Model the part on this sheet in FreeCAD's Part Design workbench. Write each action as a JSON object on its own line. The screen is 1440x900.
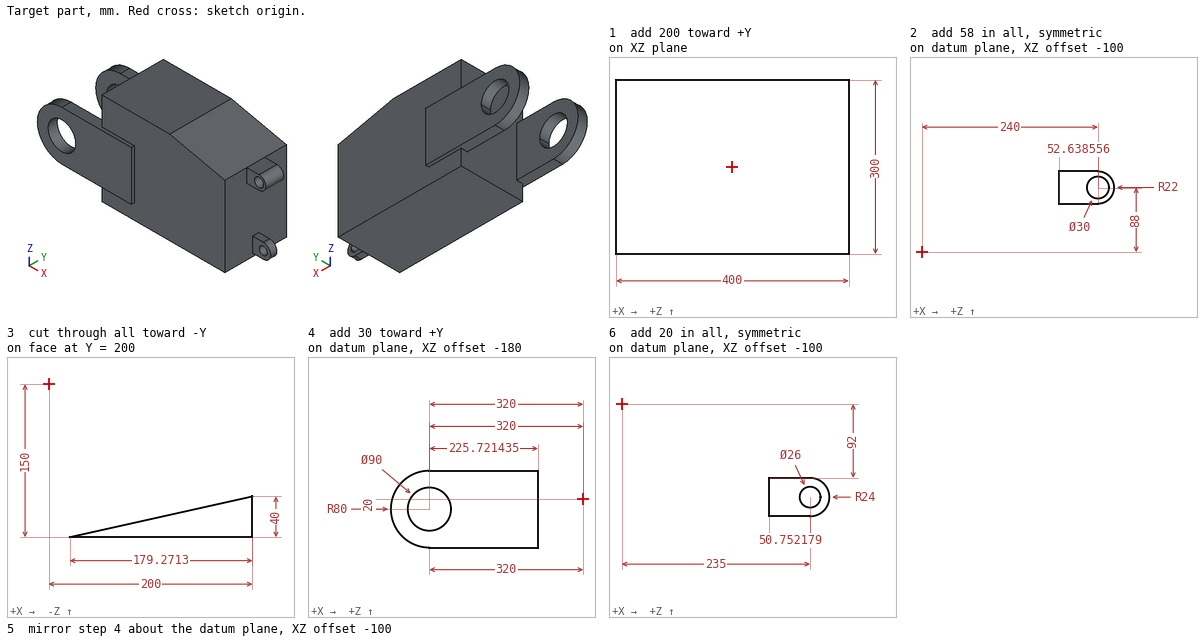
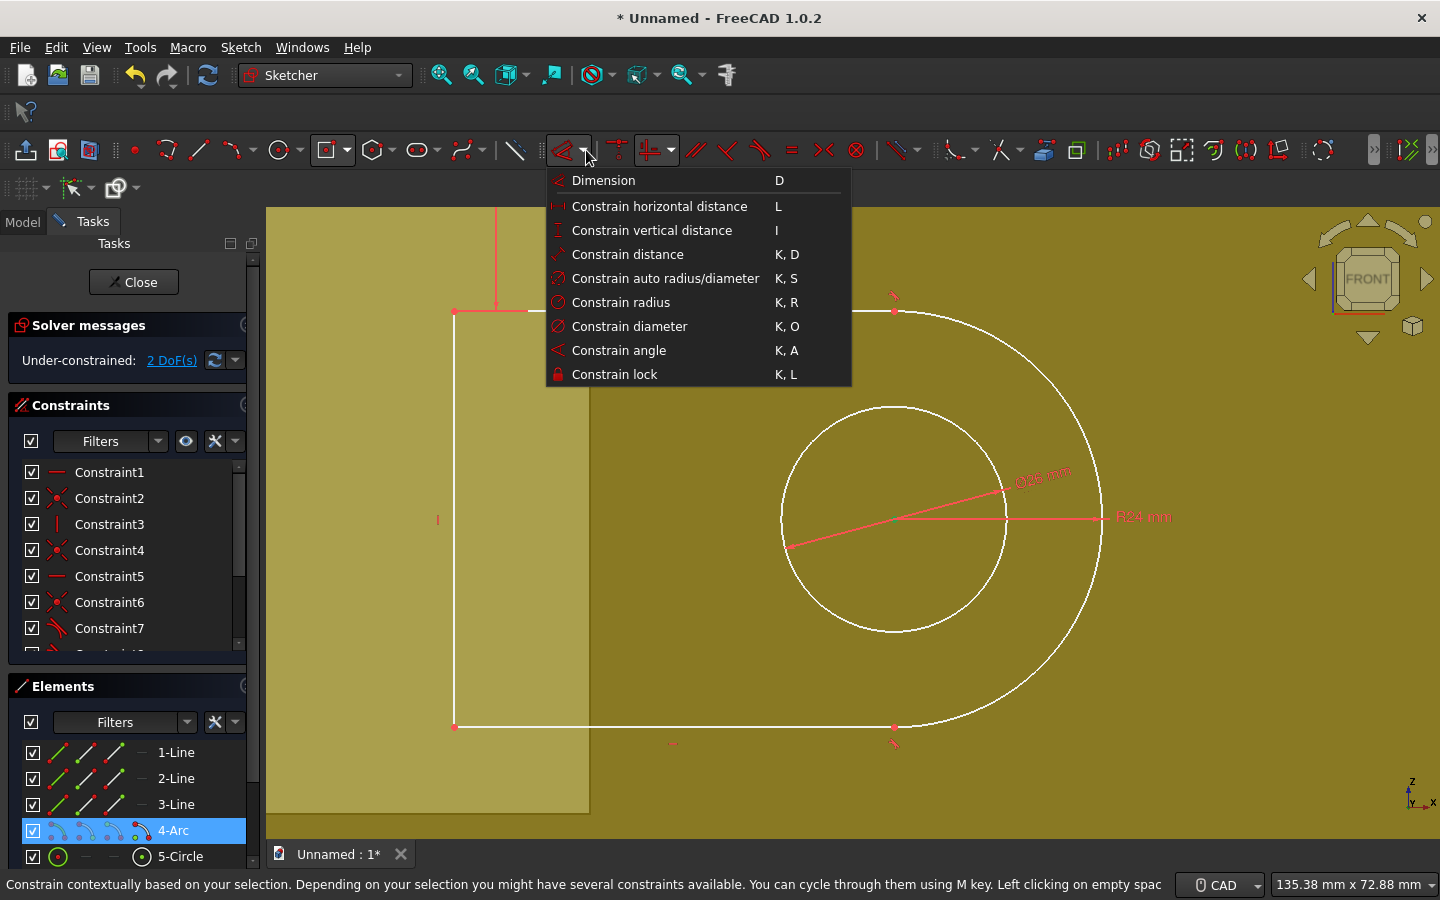
{"action": "left_click", "coordinate": [699, 206]}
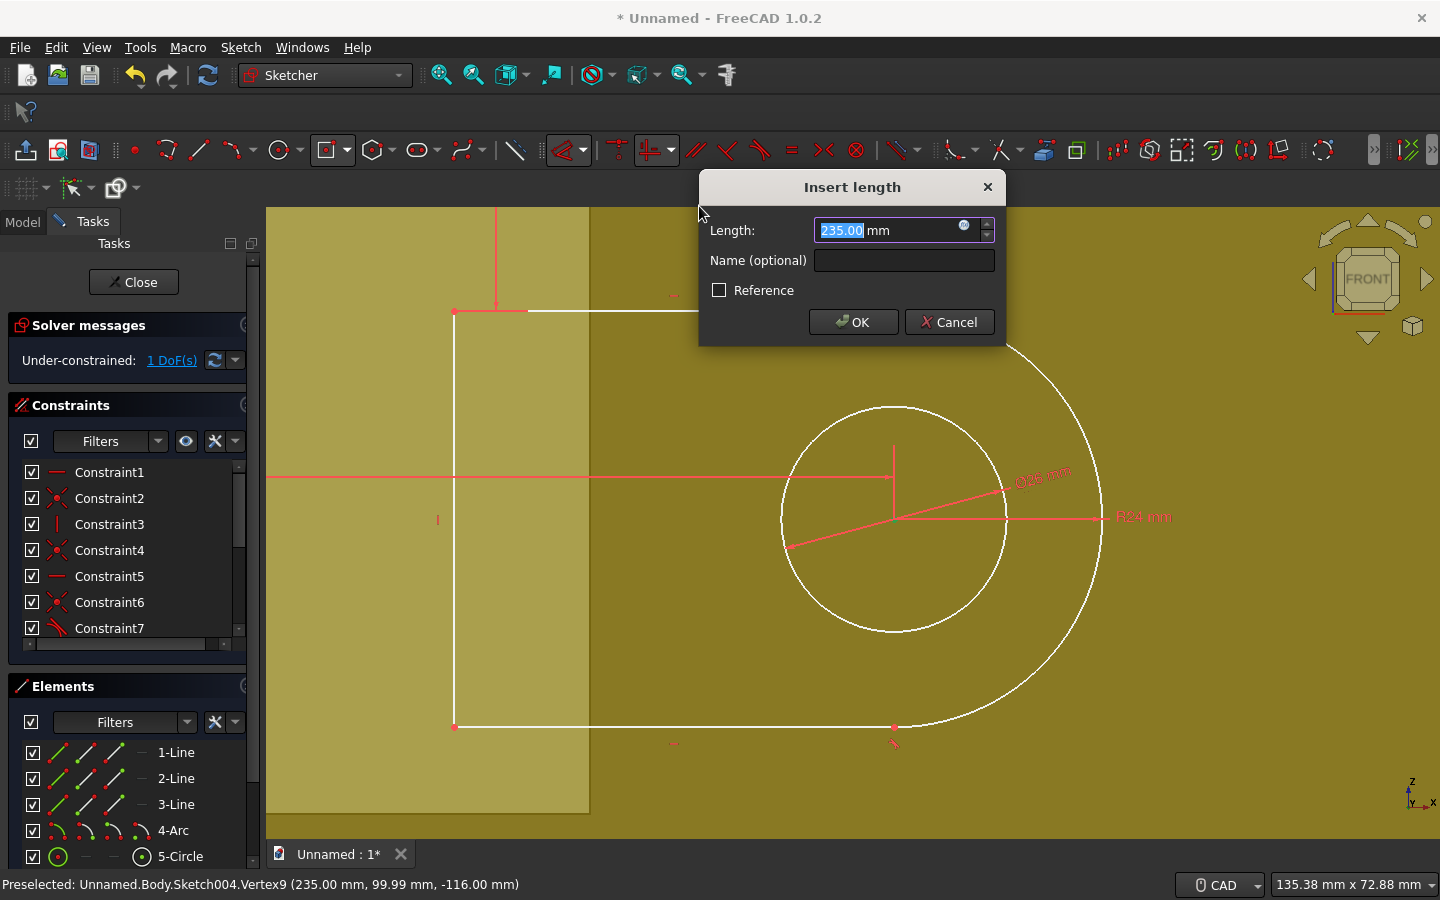
{"action": "type", "text": "235"}
{"action": "key", "text": "Return"}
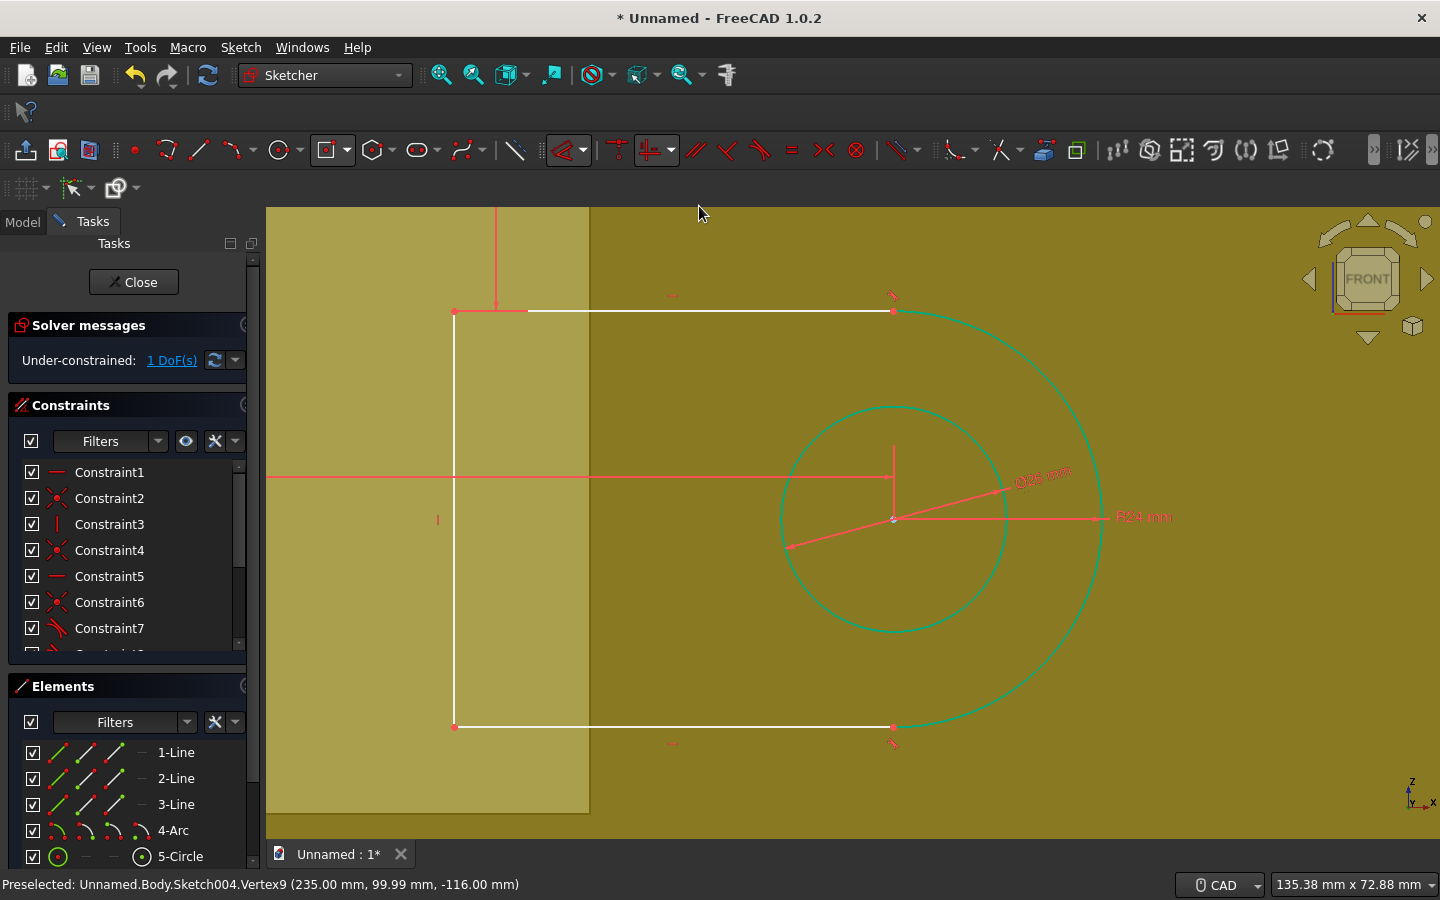
{"action": "left_click", "coordinate": [762, 727]}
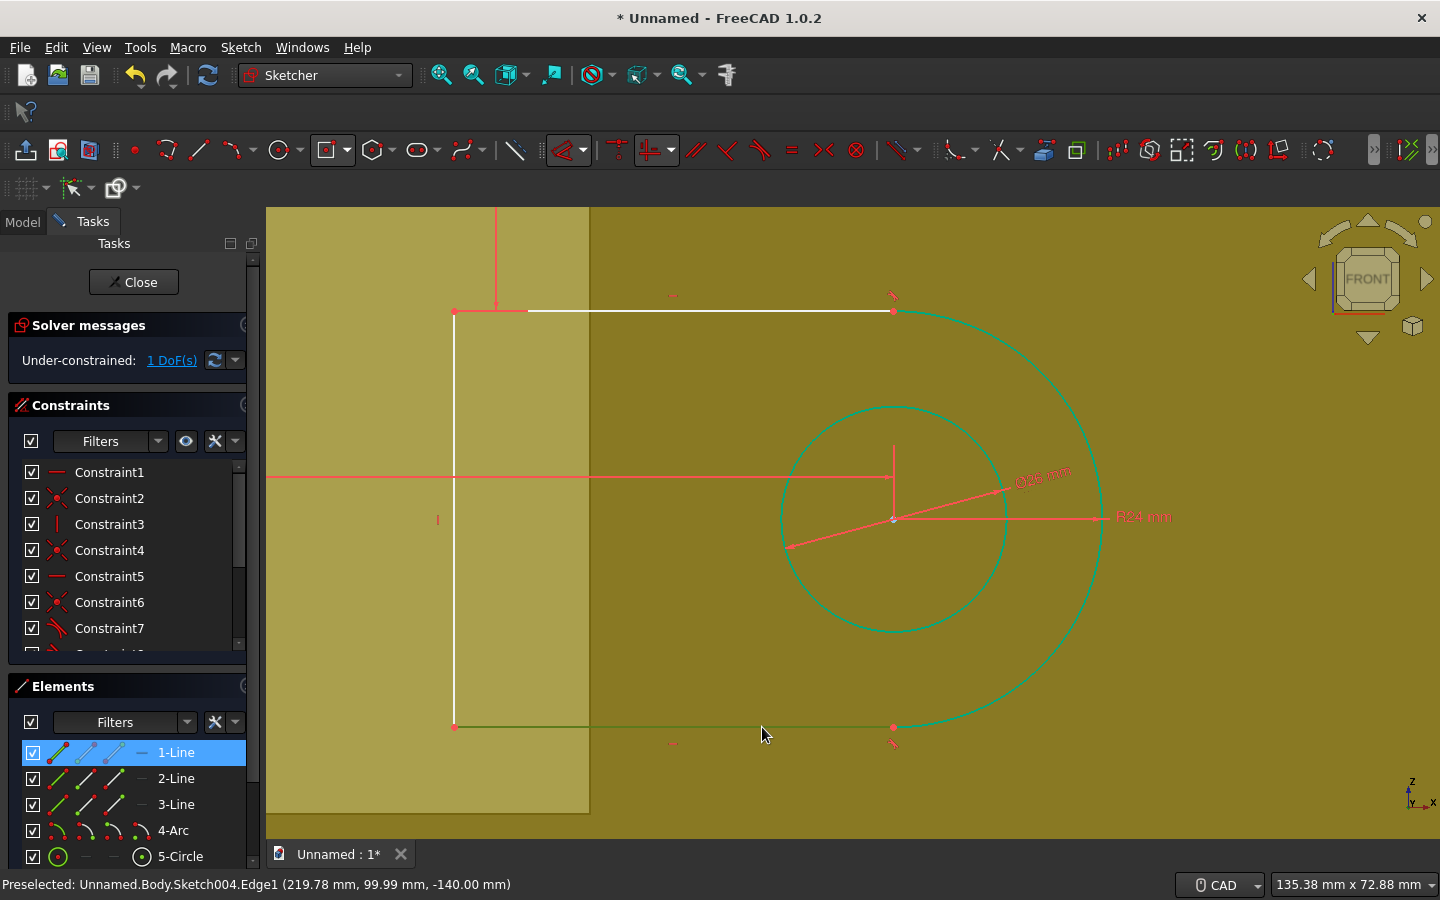
{"action": "key", "text": "l"}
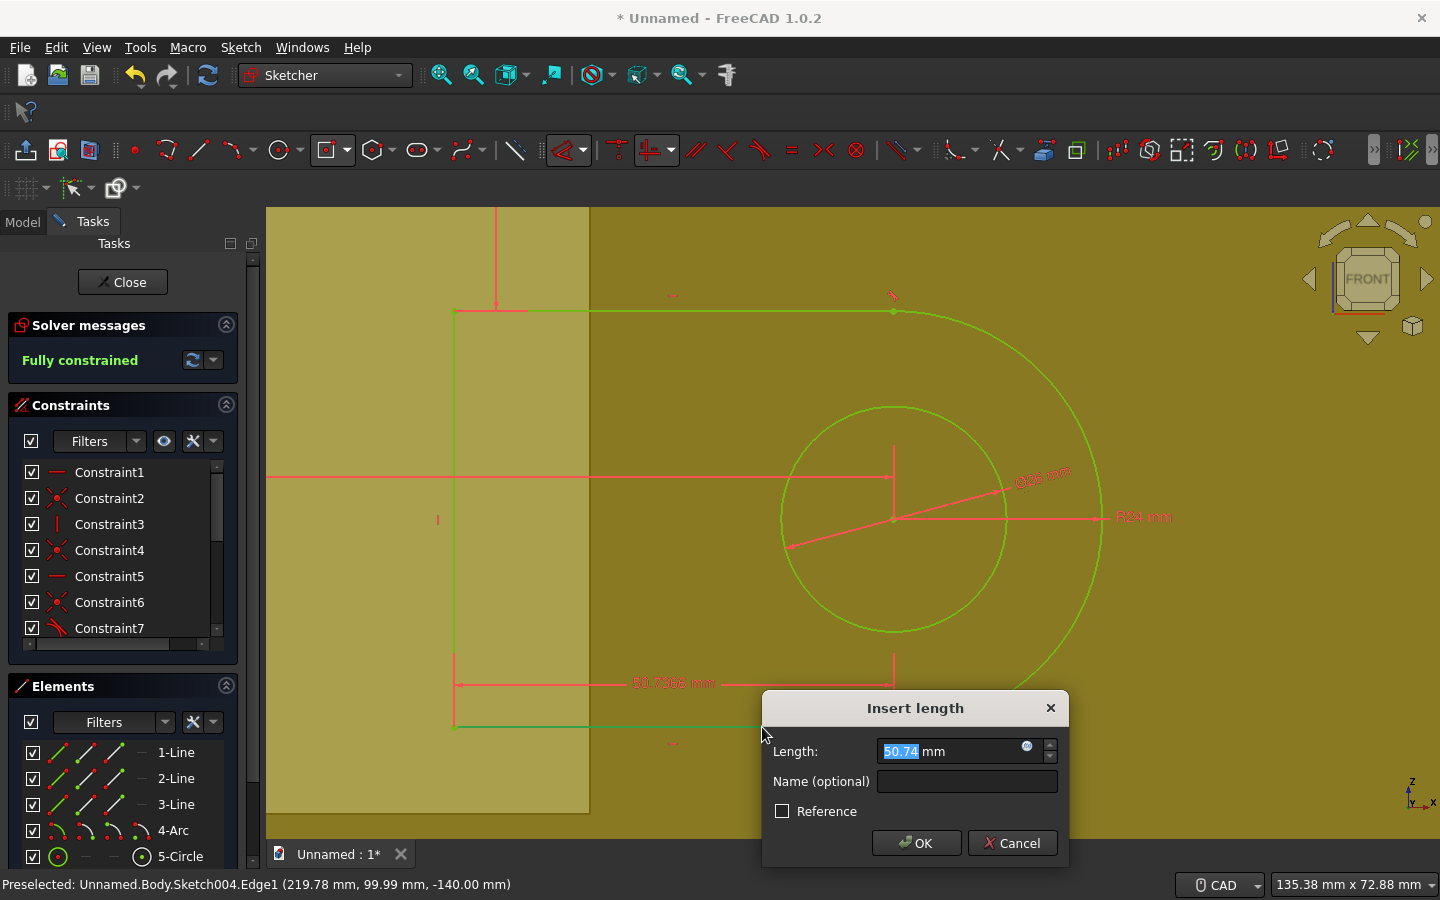
{"action": "type", "text": "50.752179"}
{"action": "key", "text": "Return"}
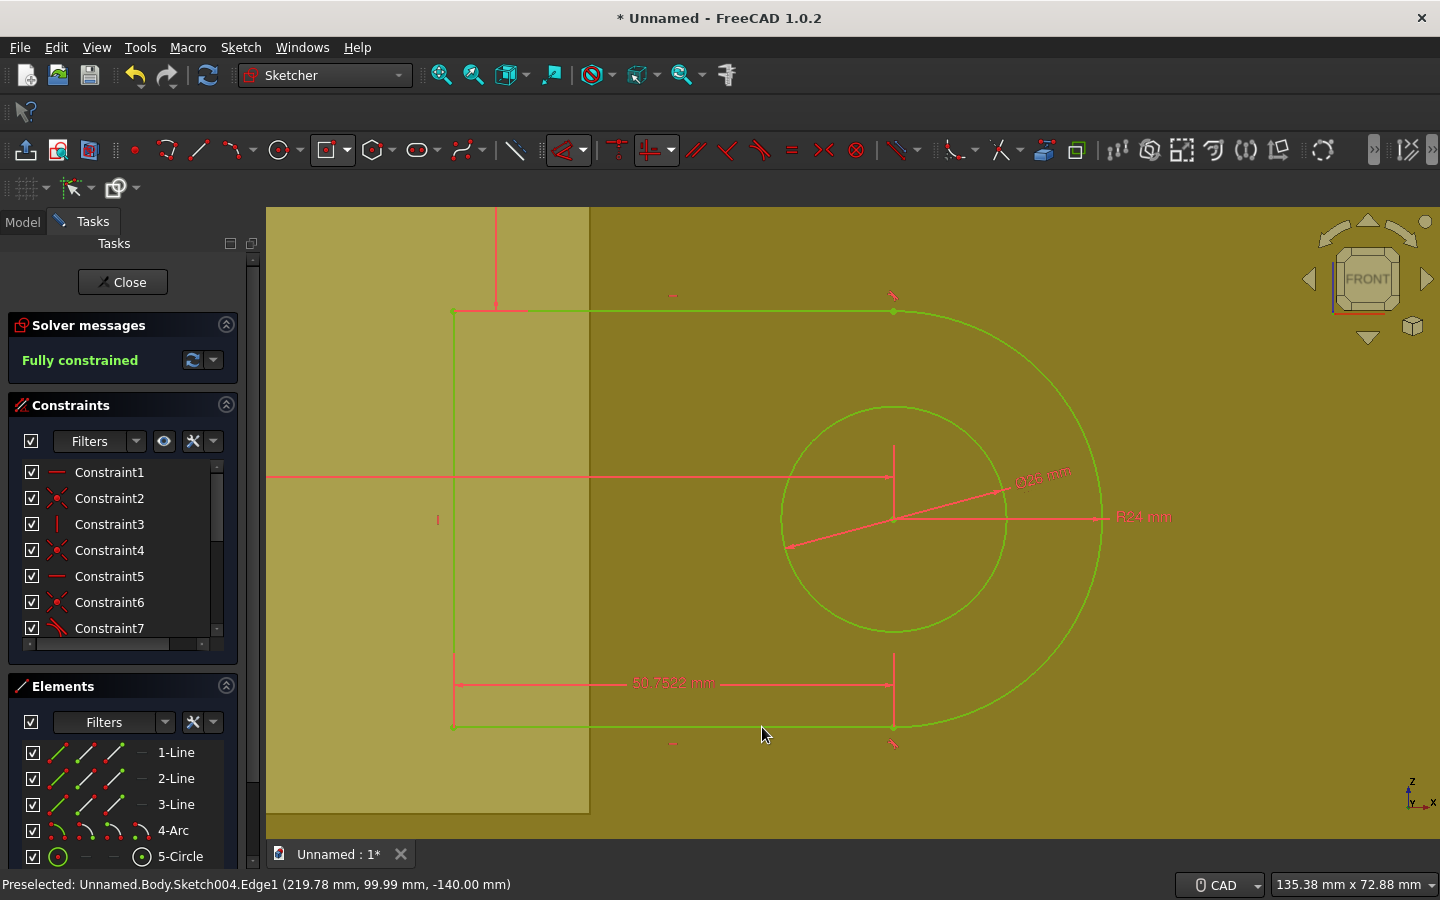
{"action": "left_click", "coordinate": [123, 282]}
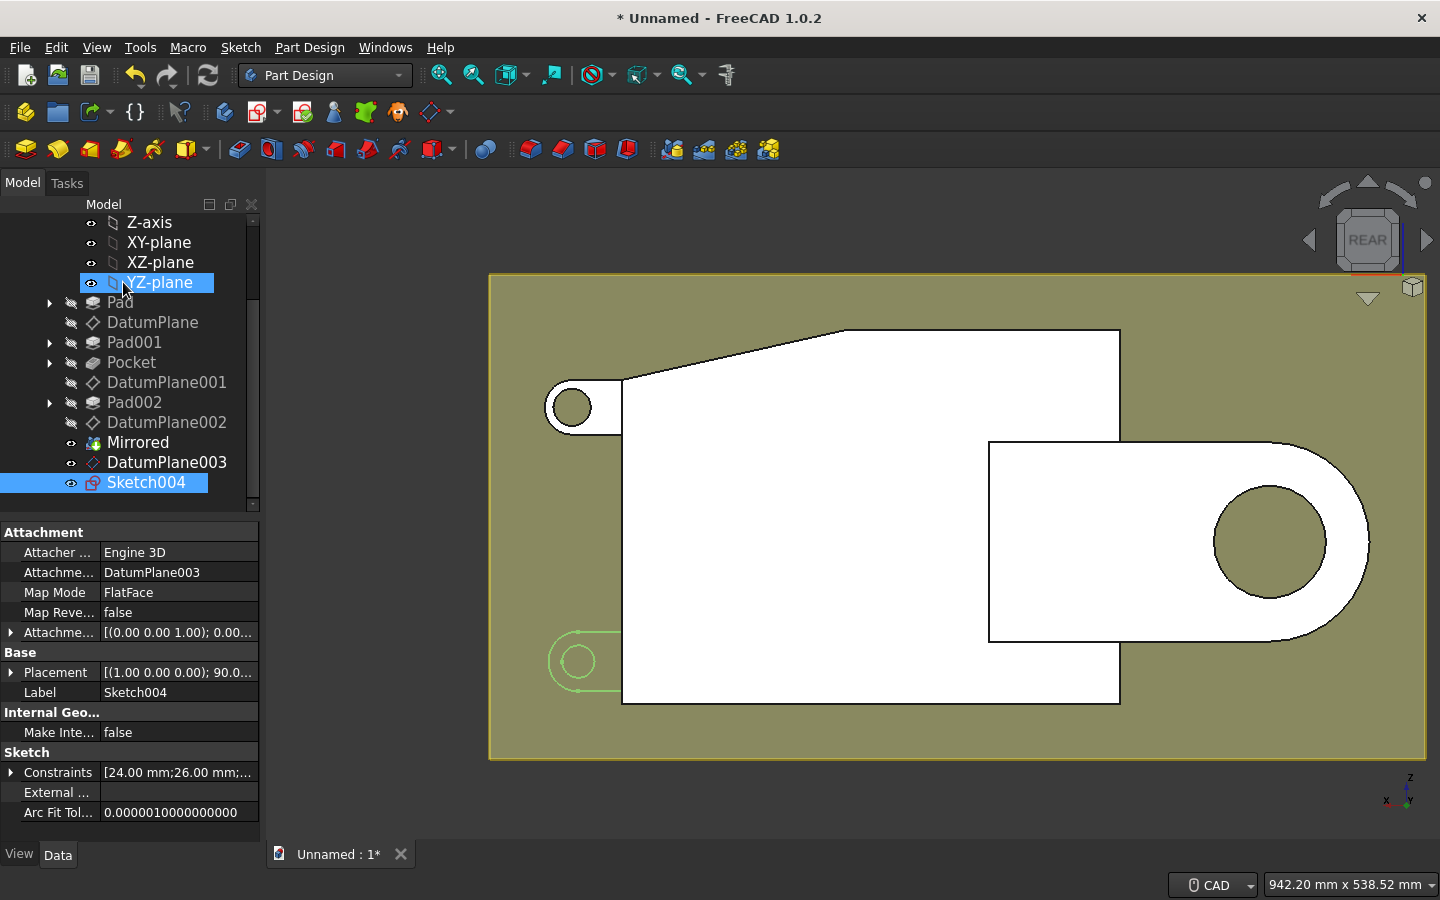
{"action": "left_click", "coordinate": [26, 150]}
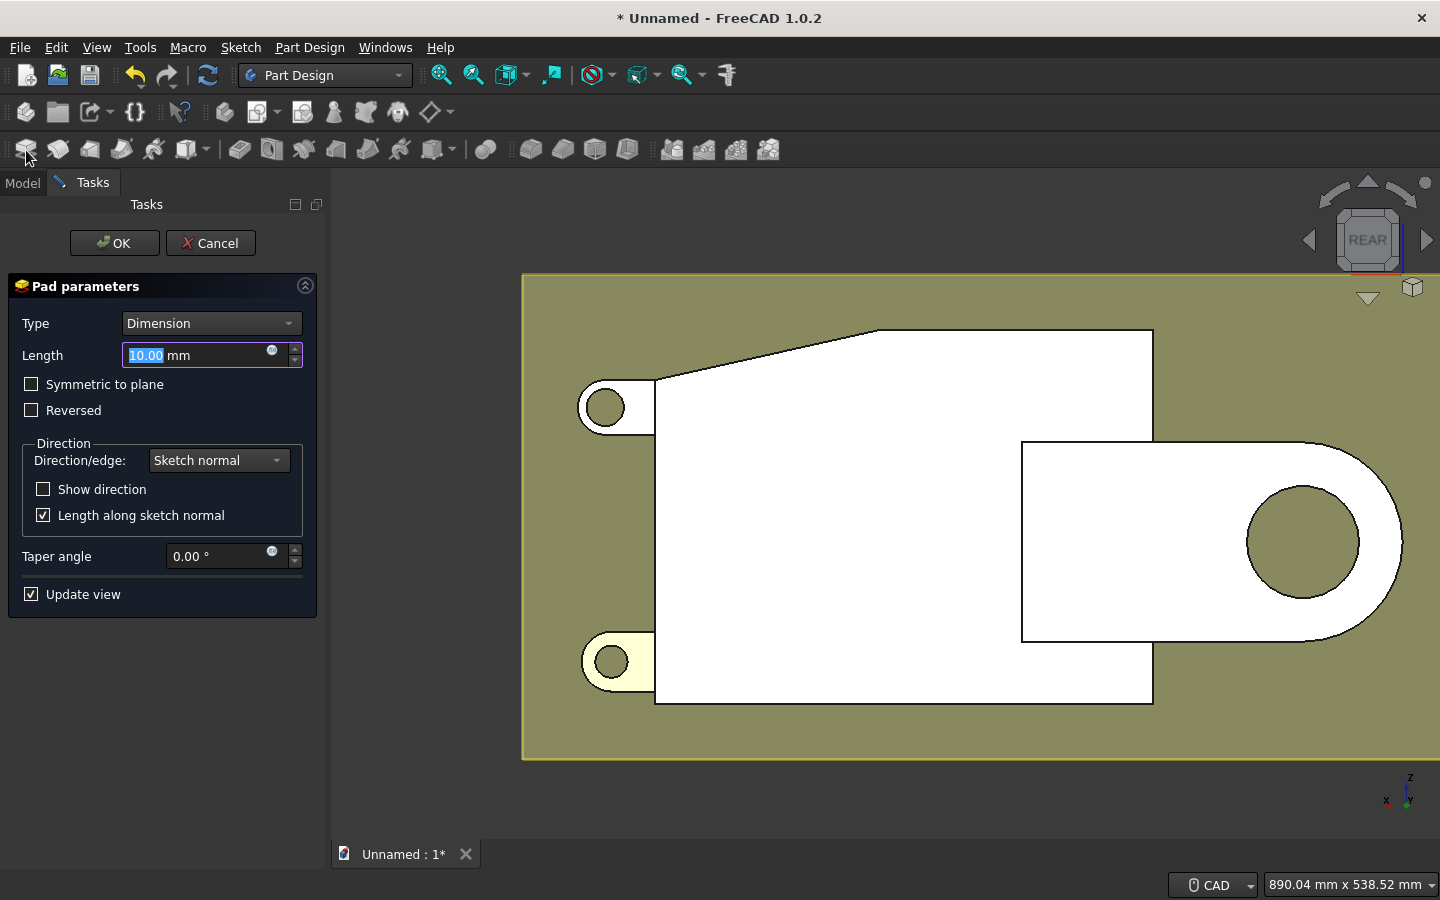
{"action": "type", "text": "20"}
{"action": "key", "text": "Tab"}